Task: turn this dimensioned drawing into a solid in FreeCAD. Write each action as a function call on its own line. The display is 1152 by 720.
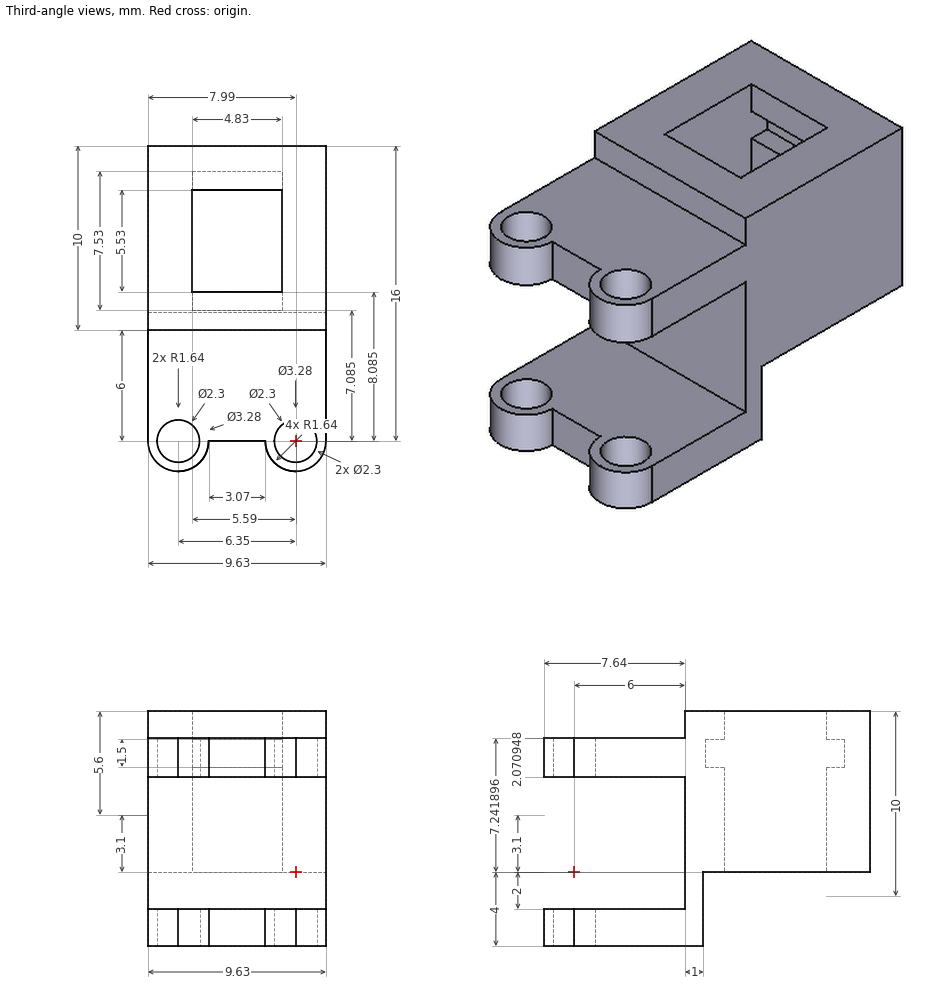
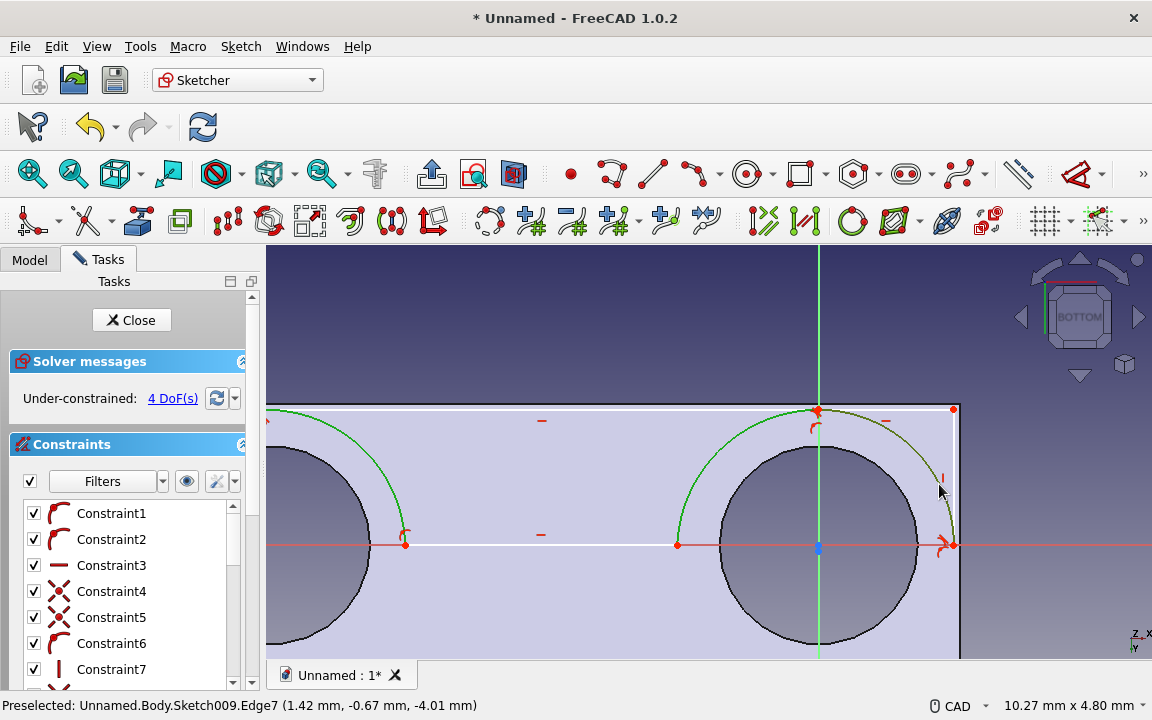
key(e)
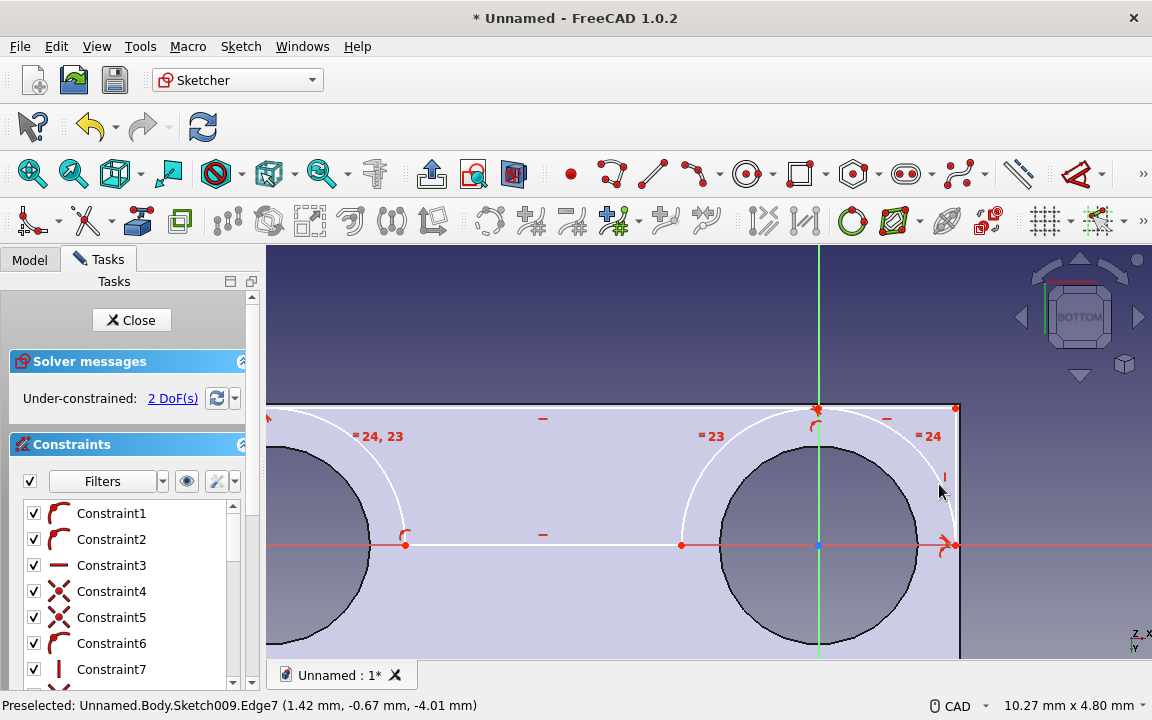
click(1076, 174)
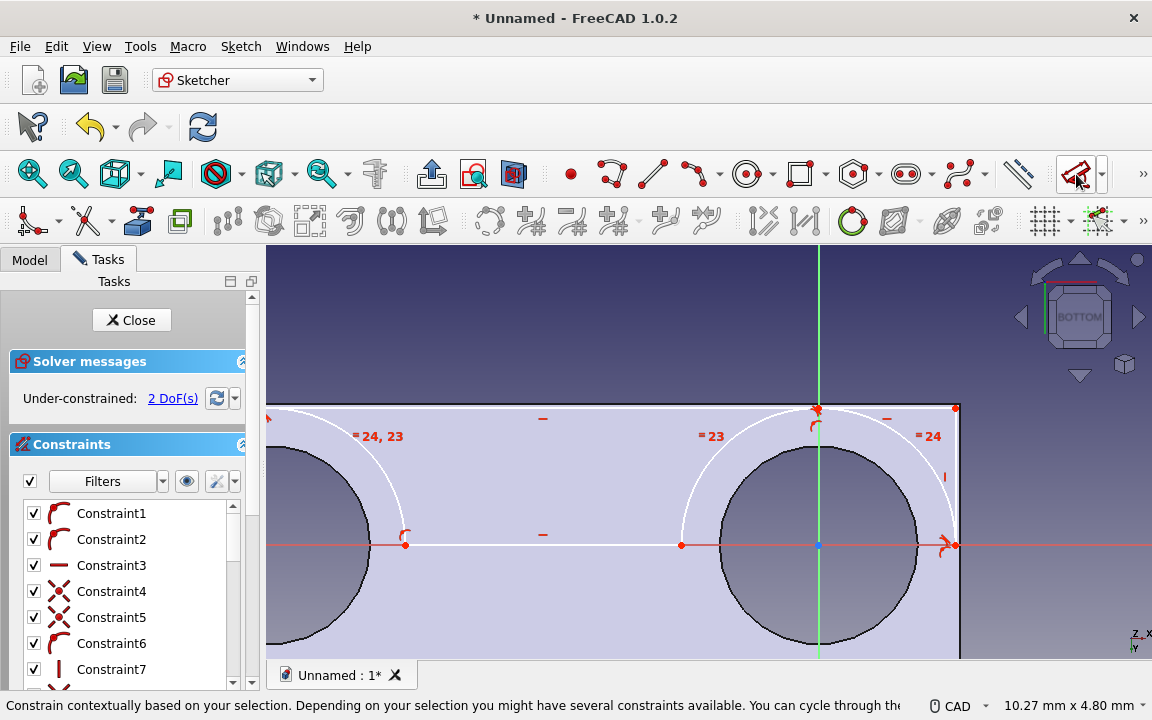
click(756, 423)
click(741, 395)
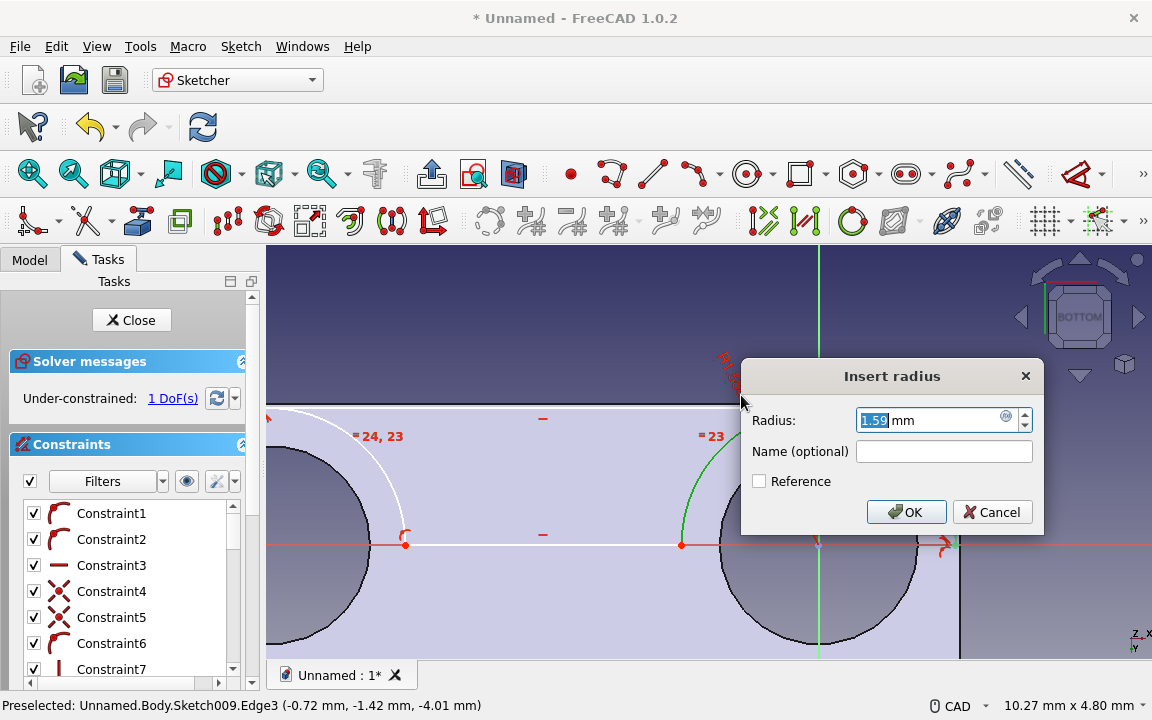
text(1.64)
key(Return)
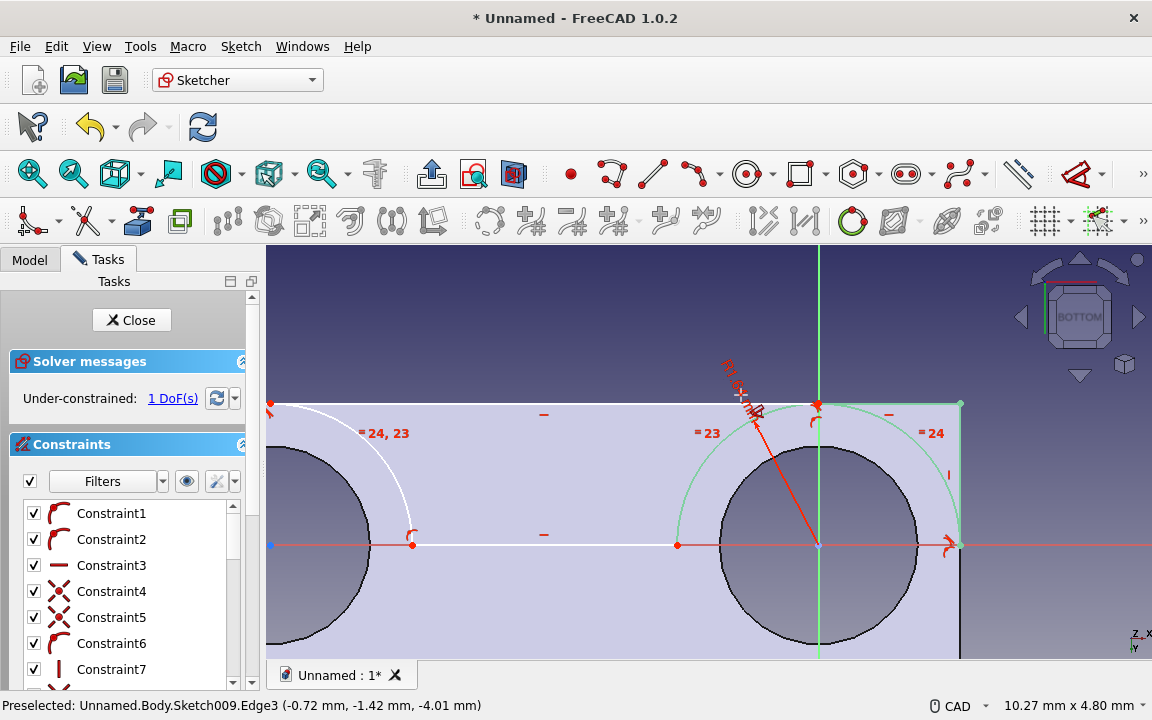
click(492, 545)
click(545, 579)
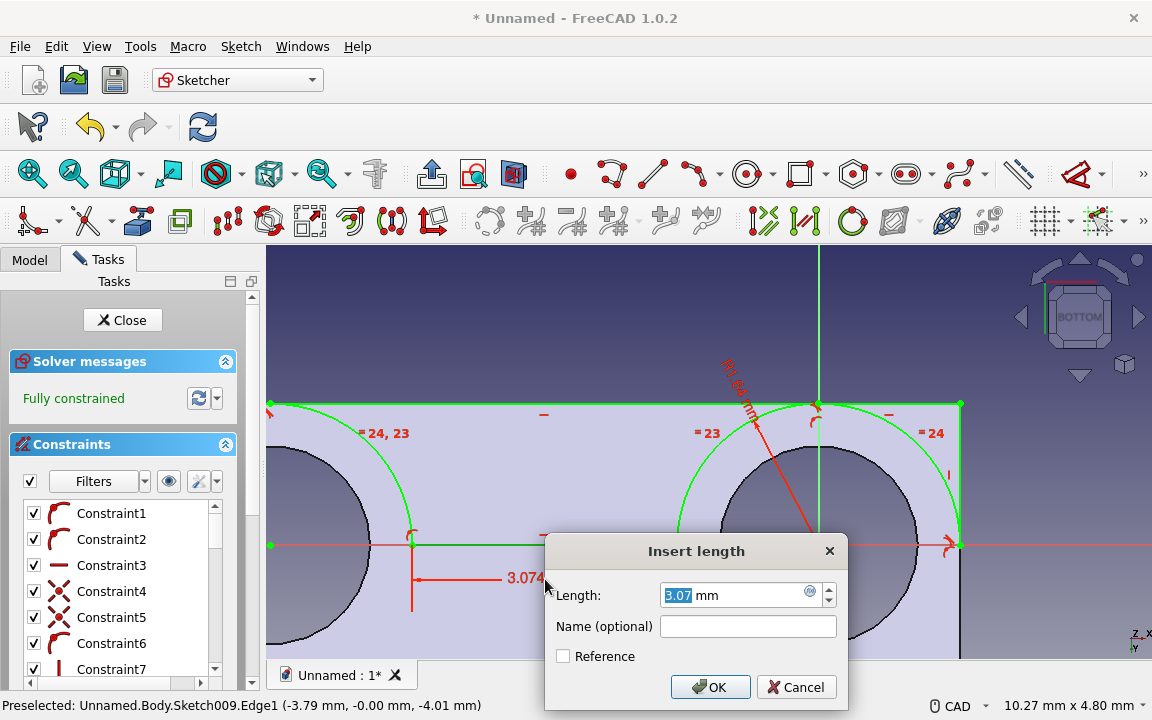
text(3.07)
key(Return)
key(Escape)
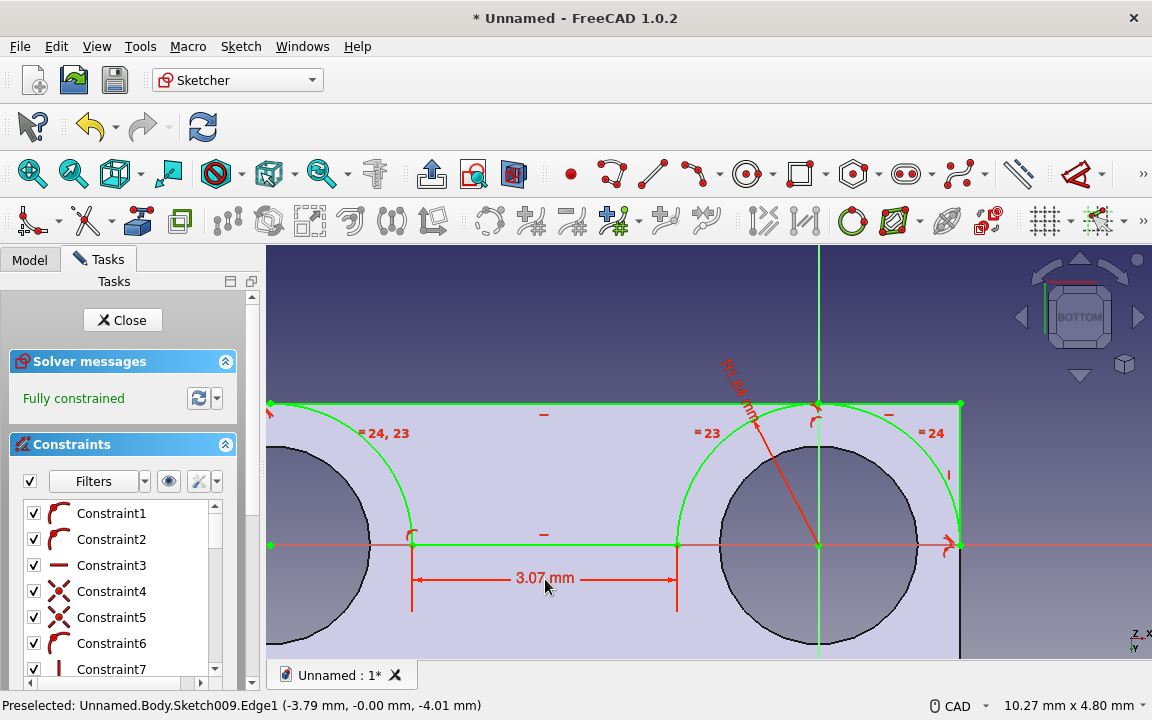
click(123, 320)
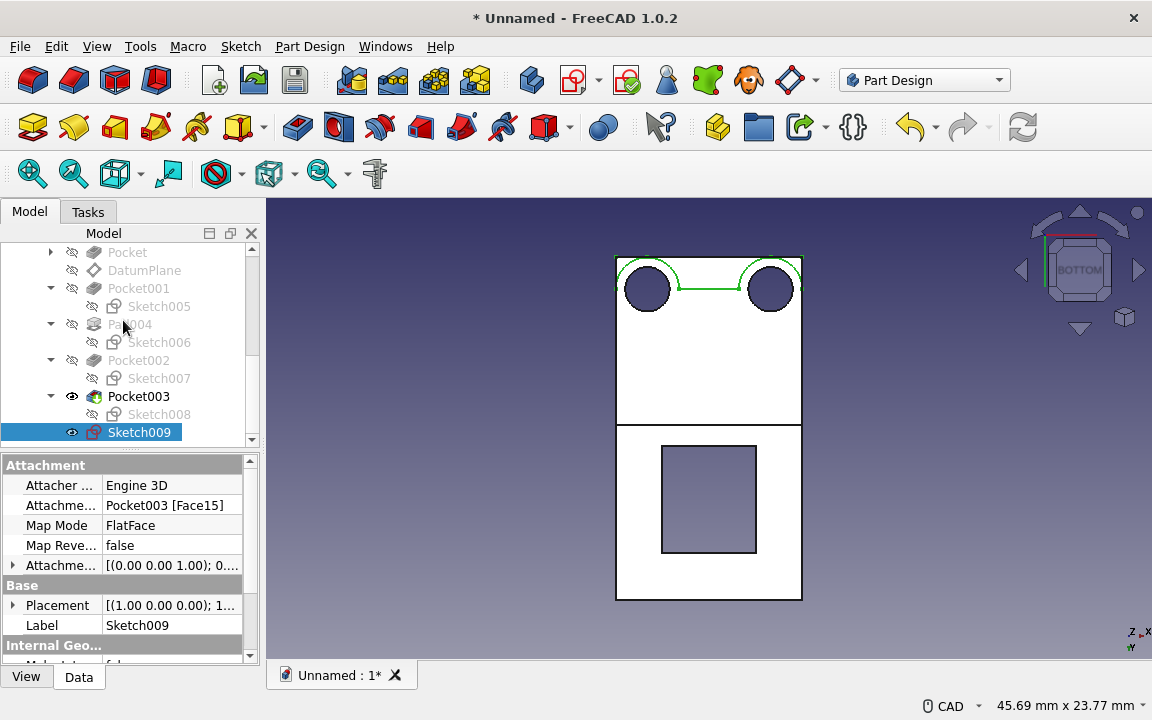
click(298, 128)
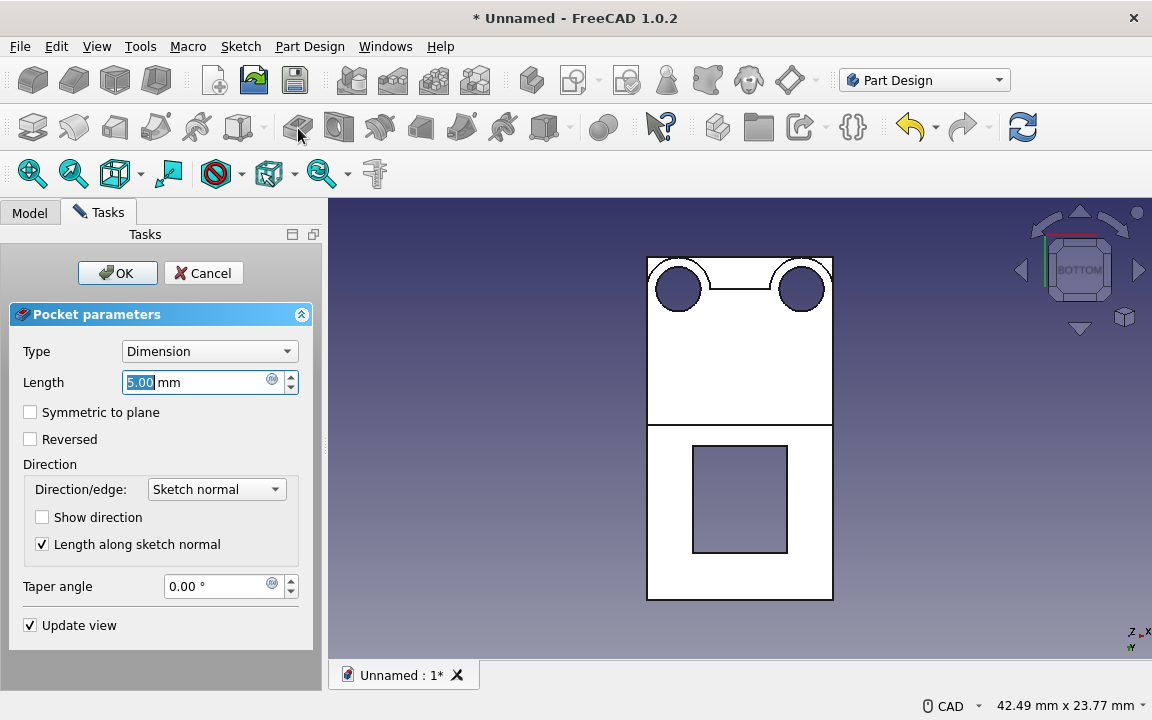
click(210, 352)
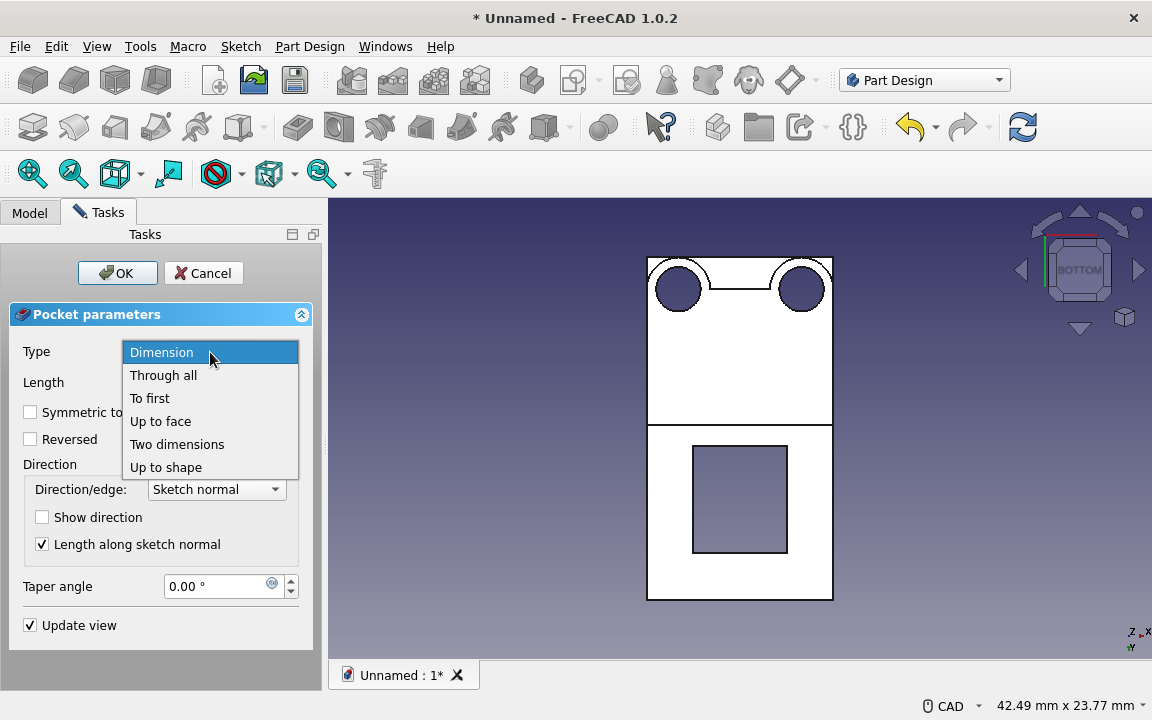
click(208, 376)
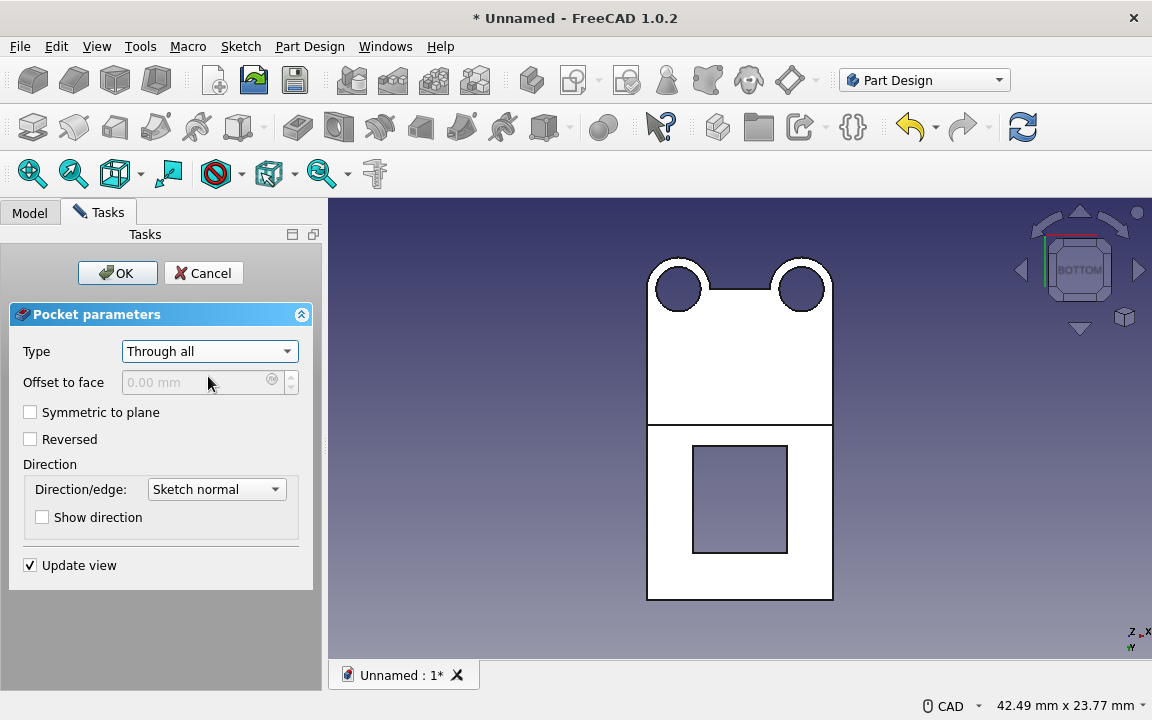
click(118, 273)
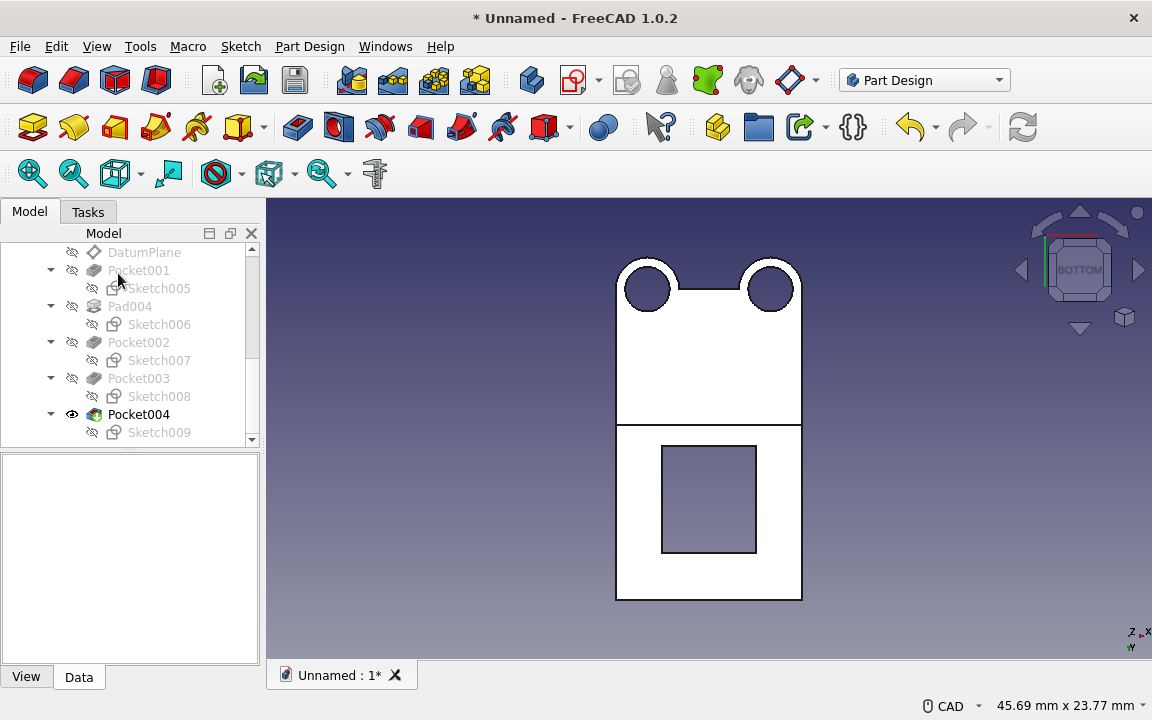
key(0)